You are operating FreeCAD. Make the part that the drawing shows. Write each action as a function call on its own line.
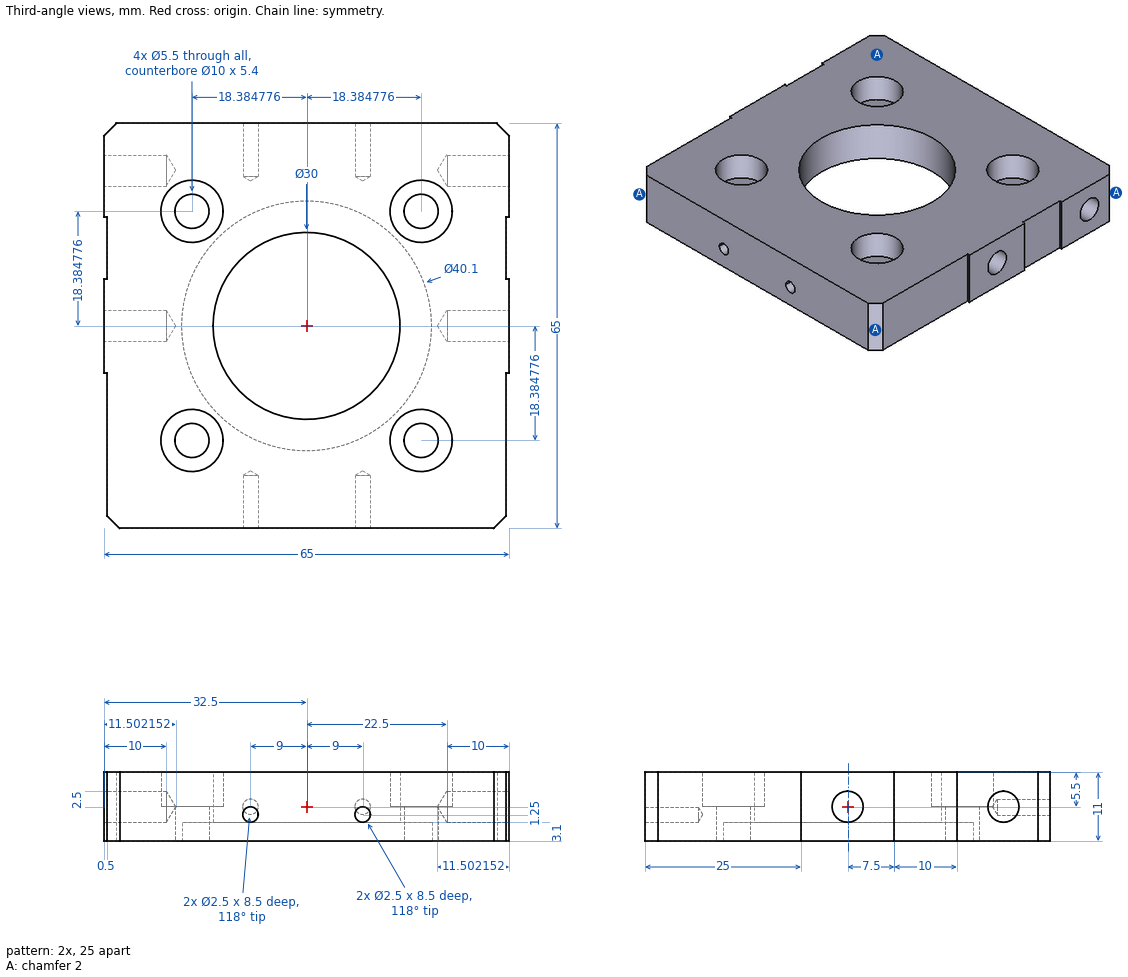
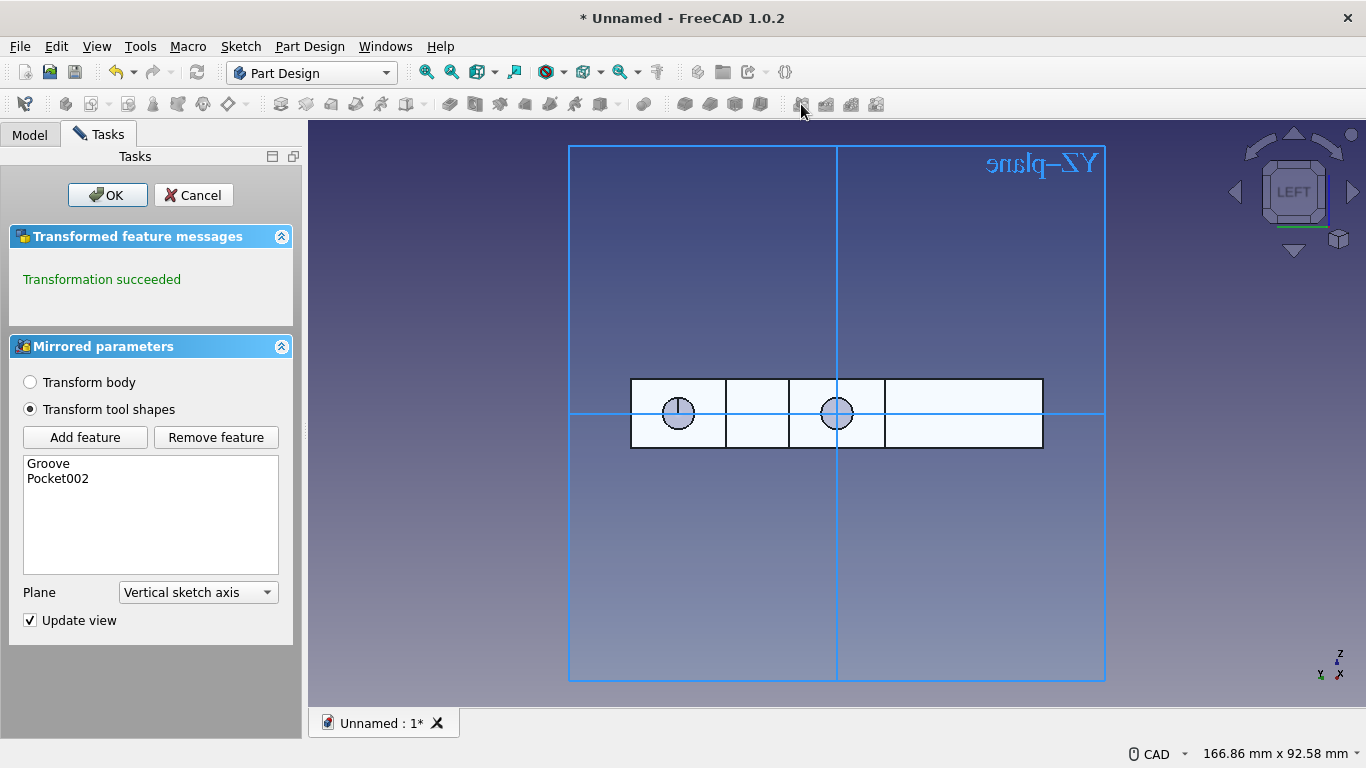
click(199, 592)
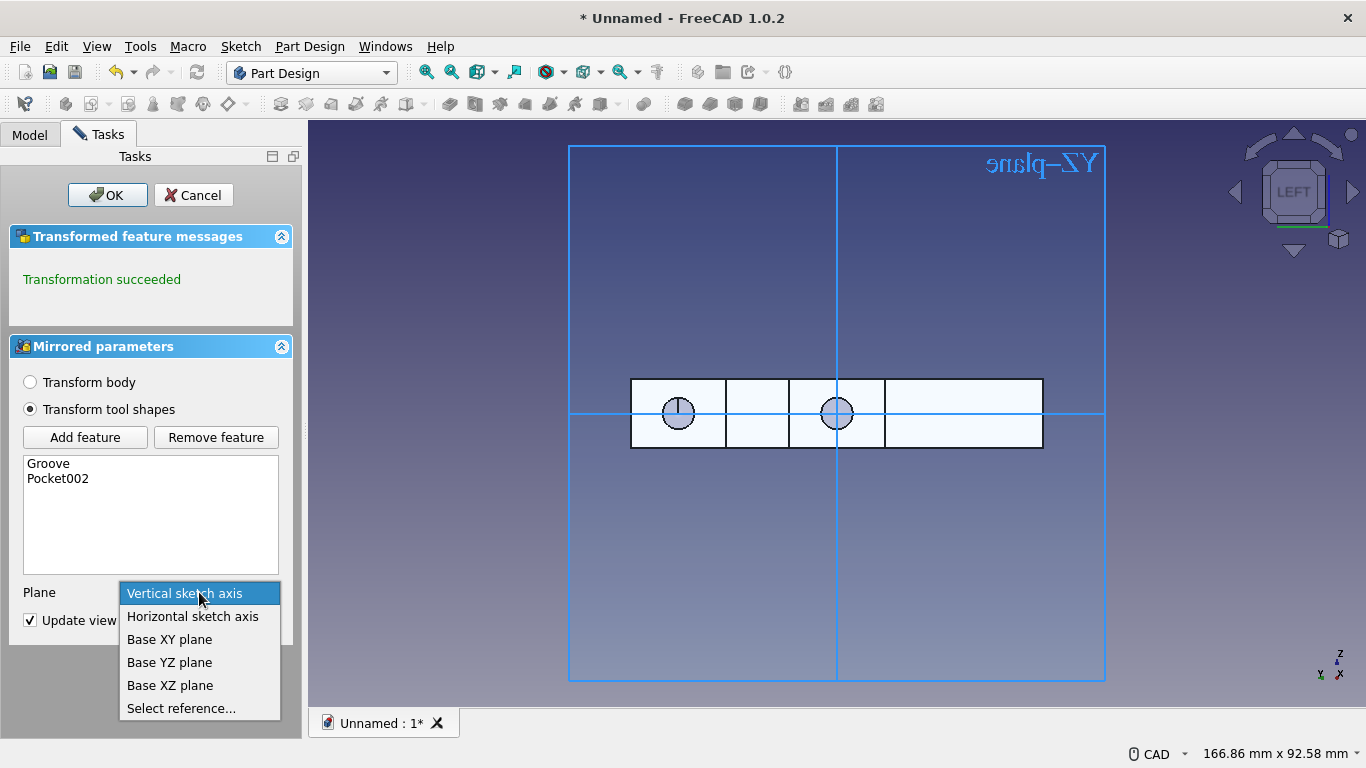
click(198, 662)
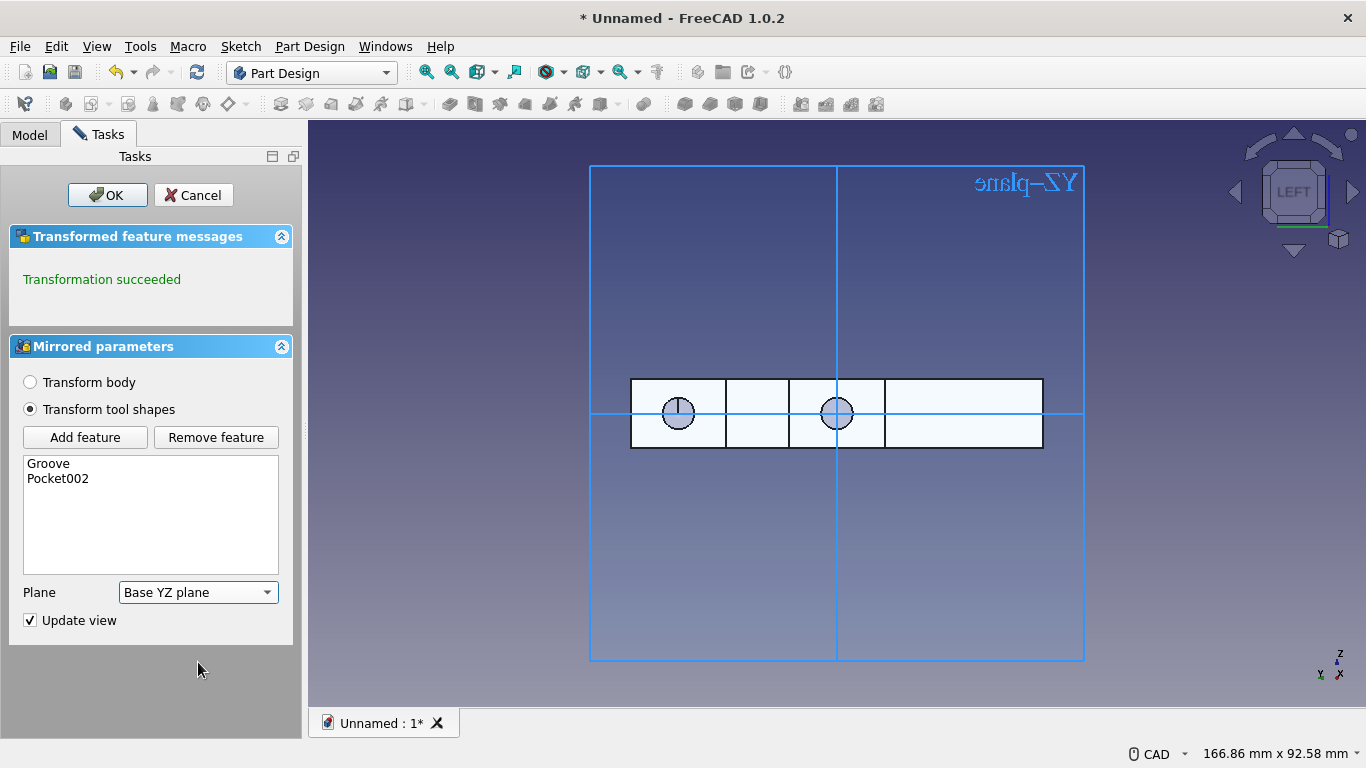
click(108, 195)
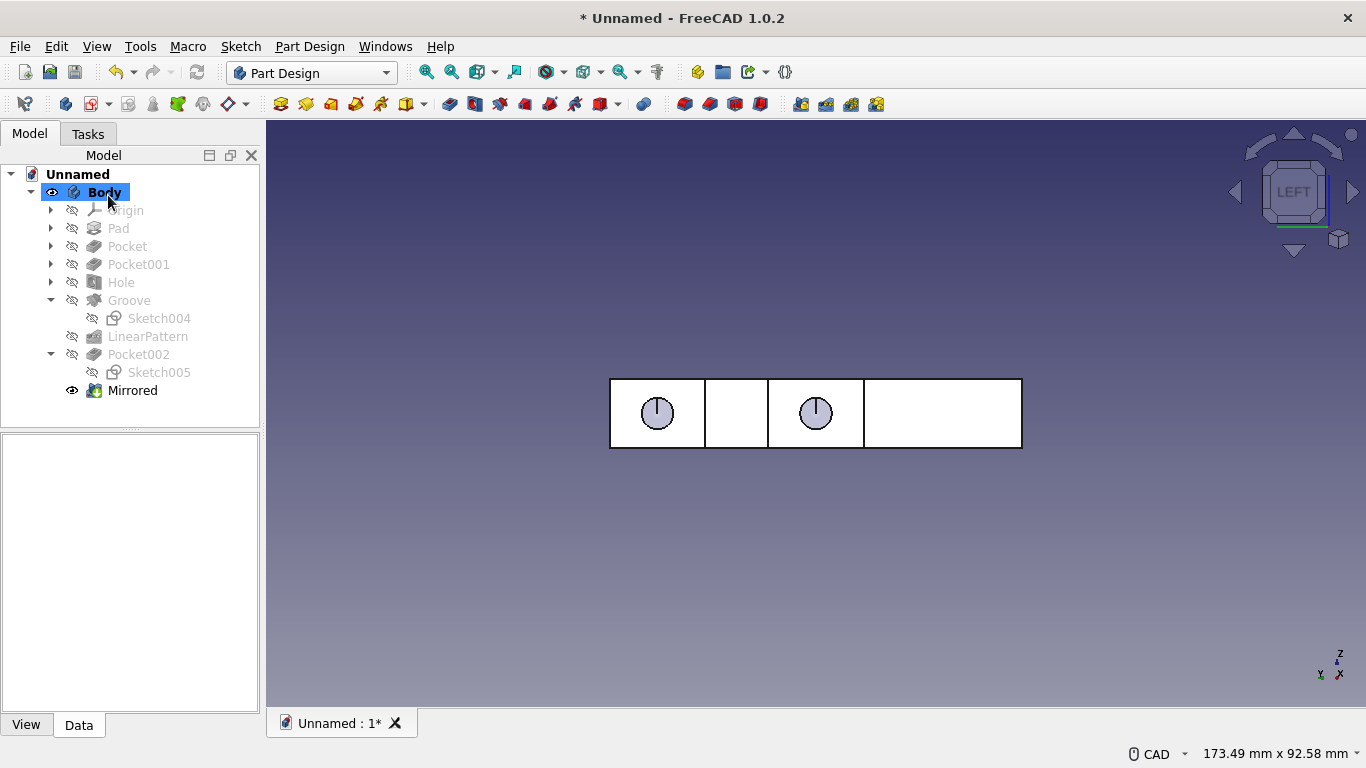
click(427, 72)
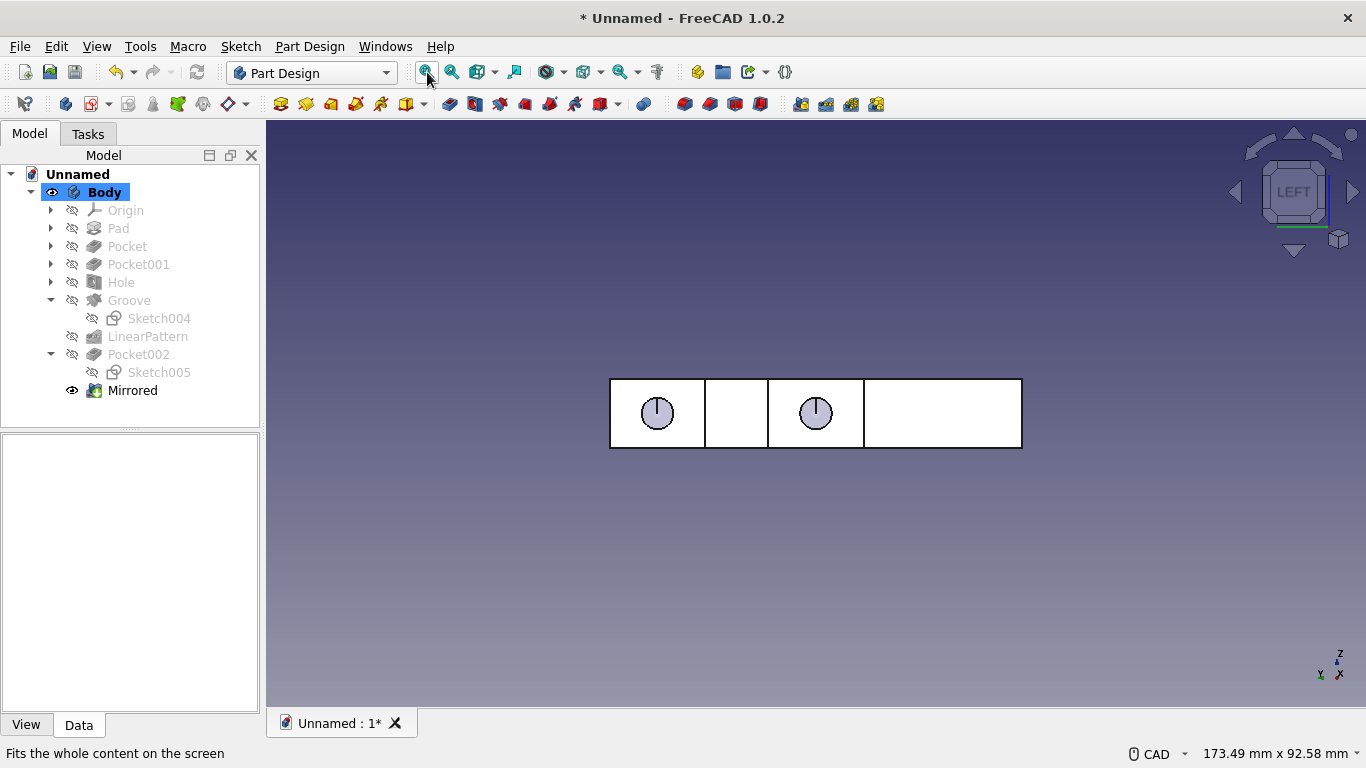
click(51, 210)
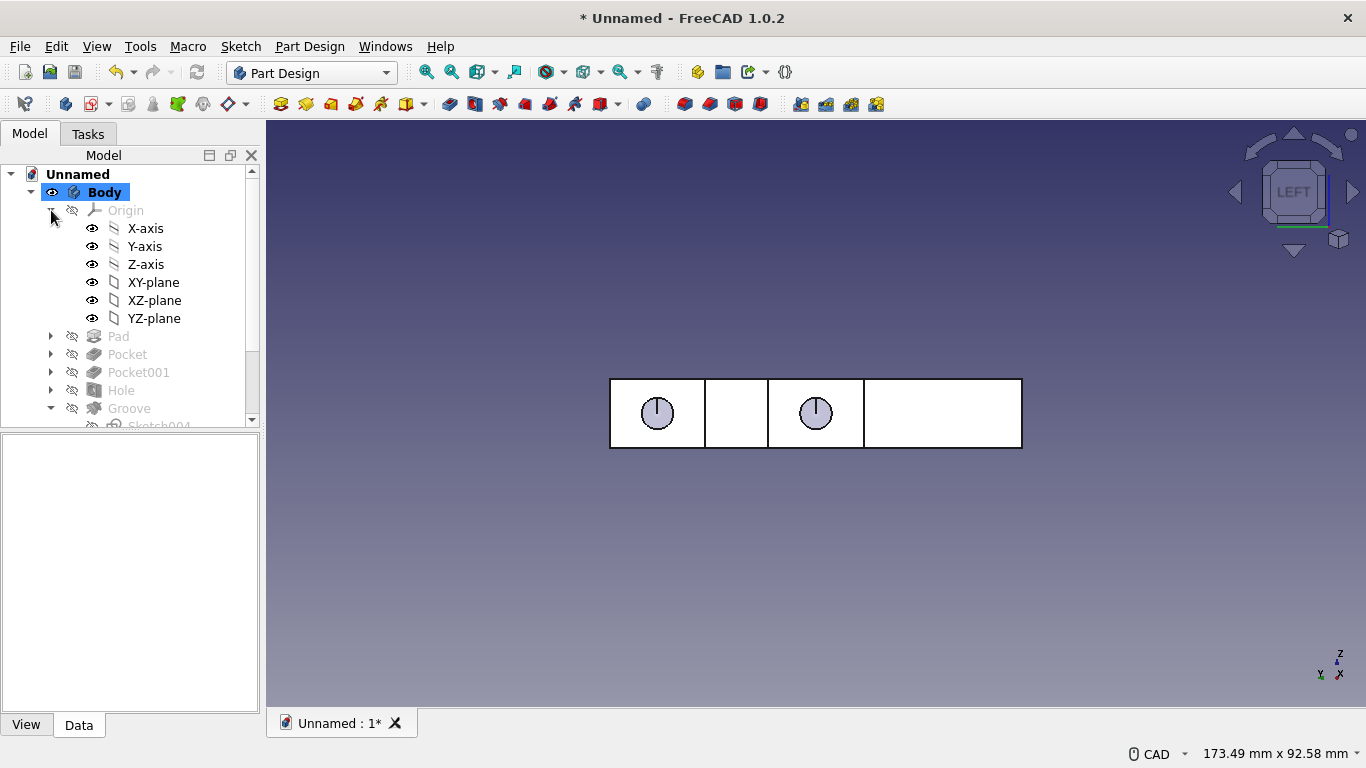
click(137, 300)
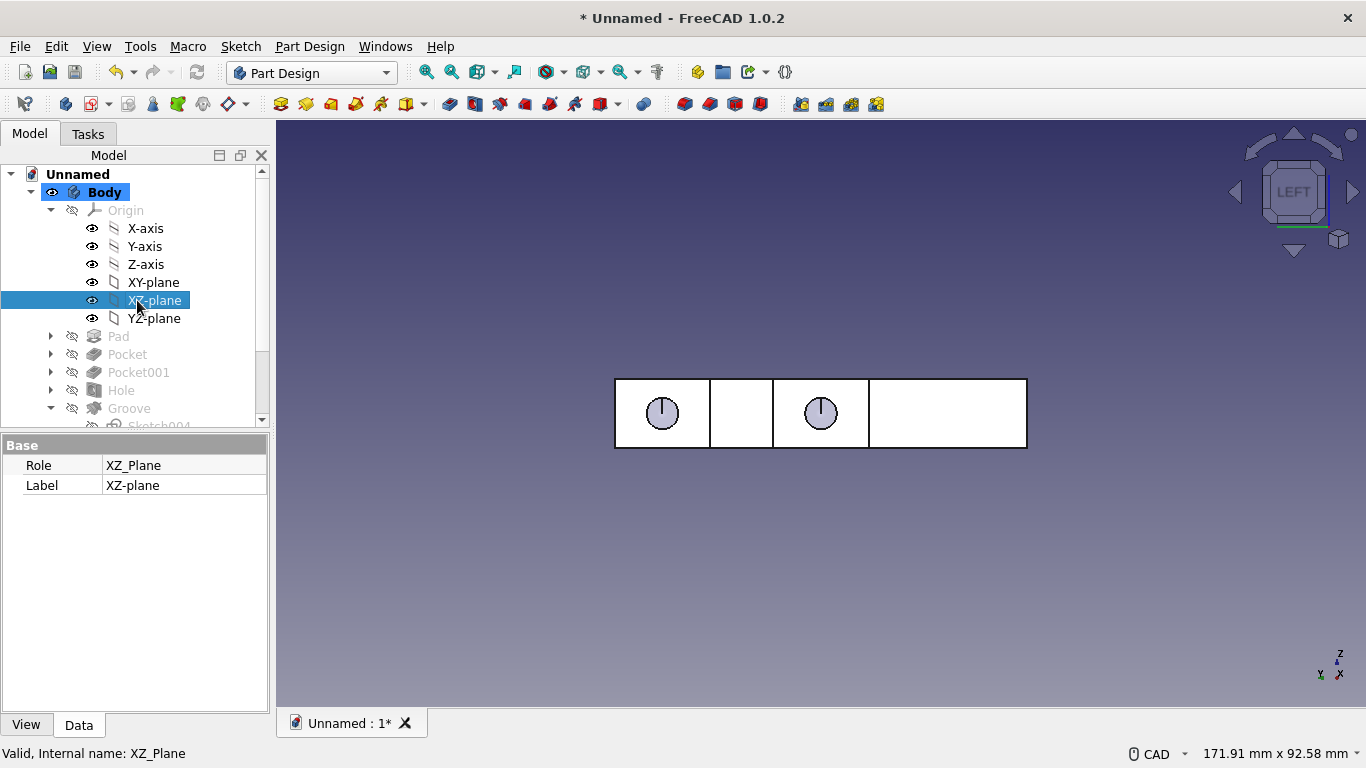
click(228, 104)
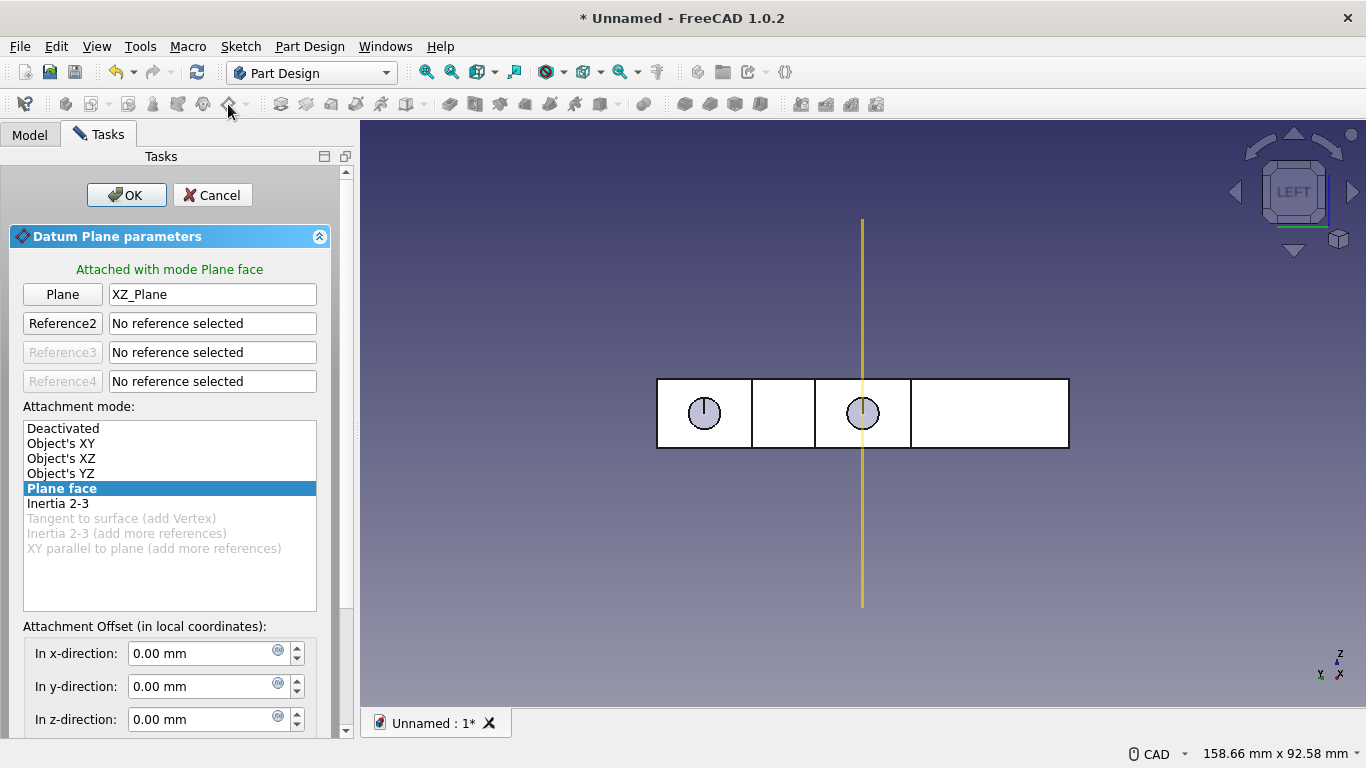
triple_click(210, 720)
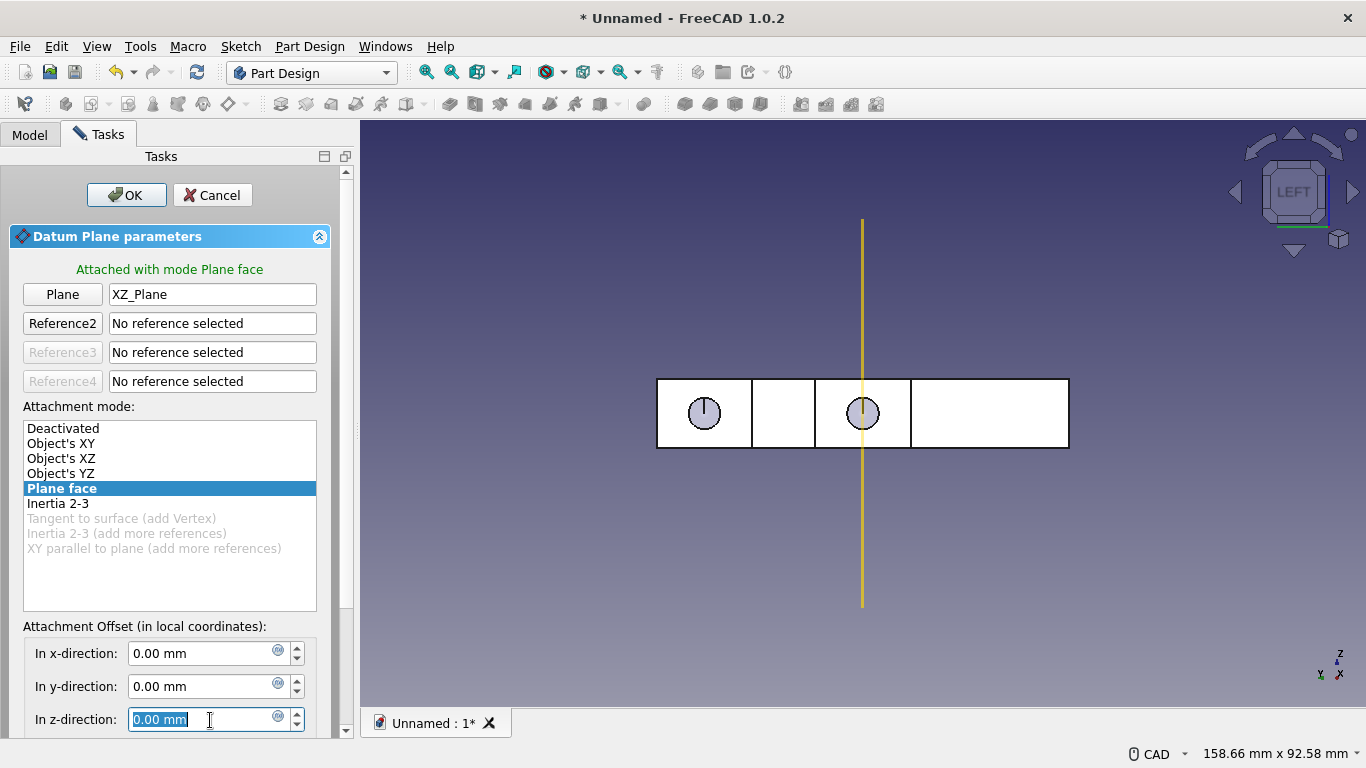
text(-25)
key(Tab)